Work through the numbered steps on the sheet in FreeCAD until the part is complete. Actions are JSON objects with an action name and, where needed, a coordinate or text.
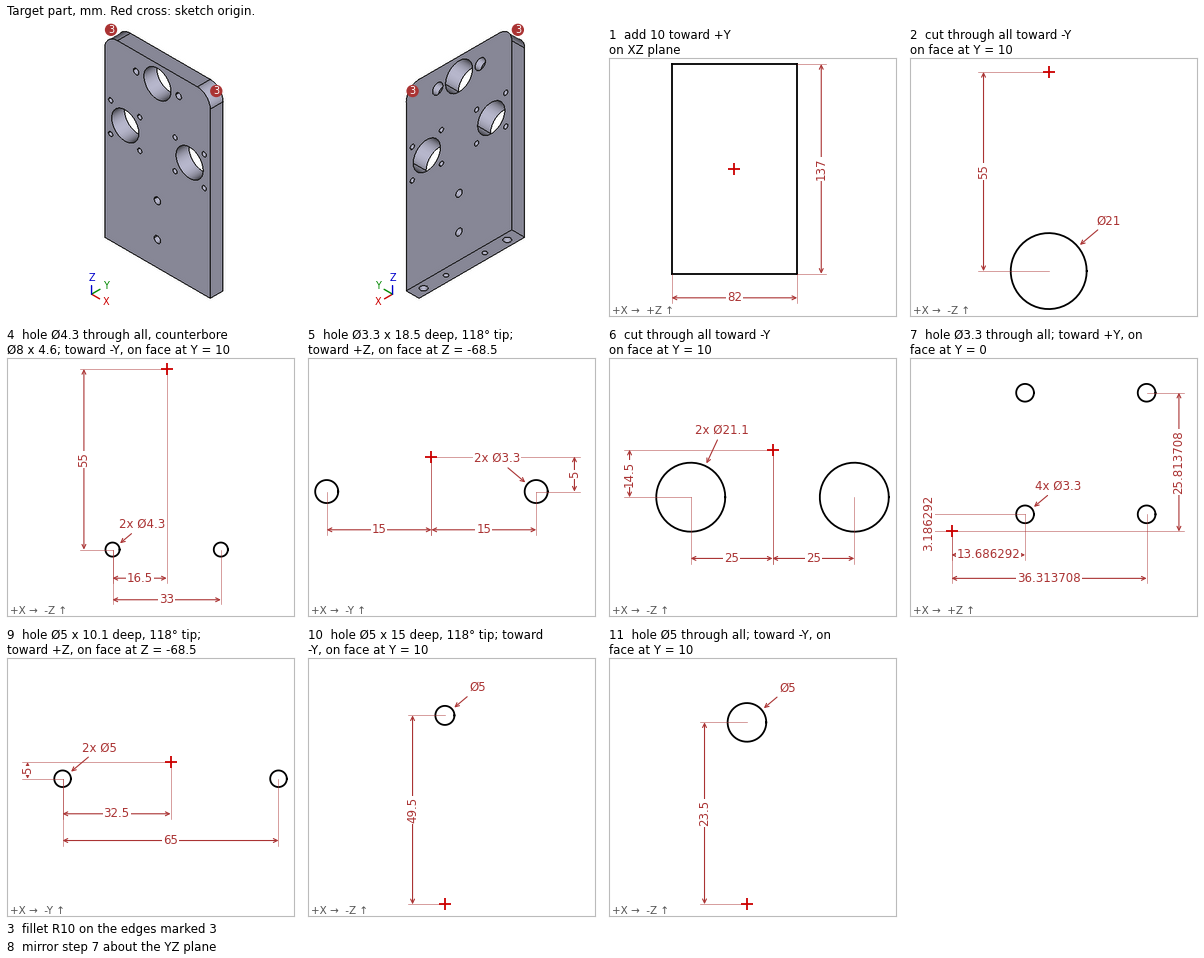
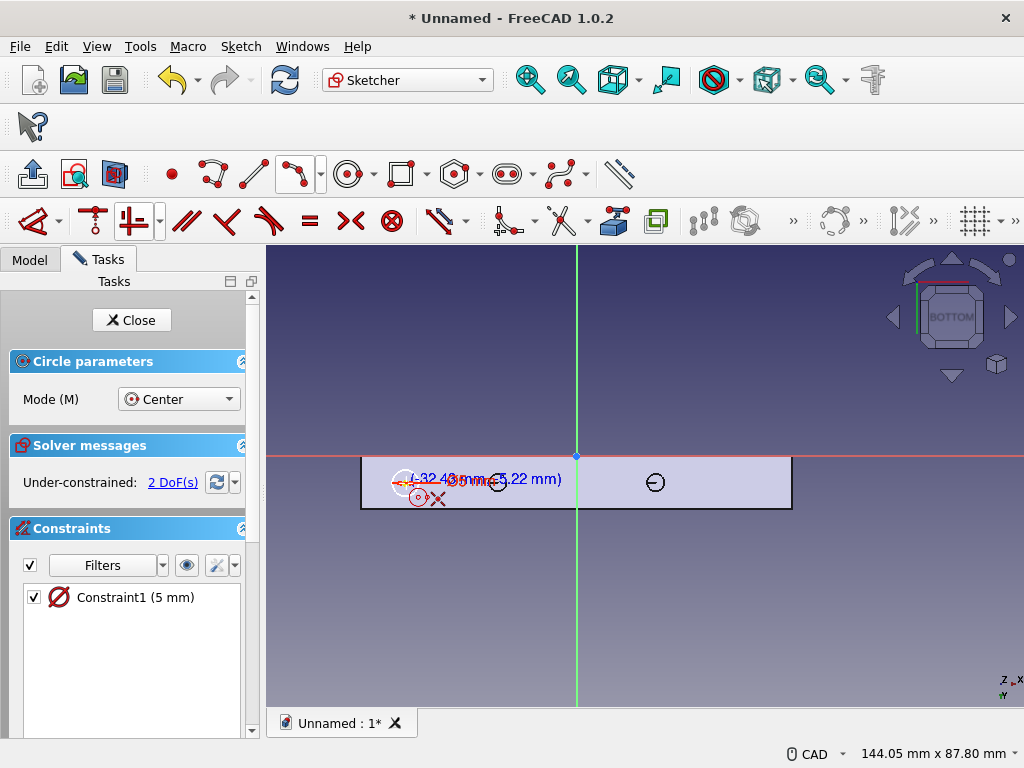
{"action": "scroll", "coordinate": [748, 483], "scroll_direction": "up", "scroll_amount": 3}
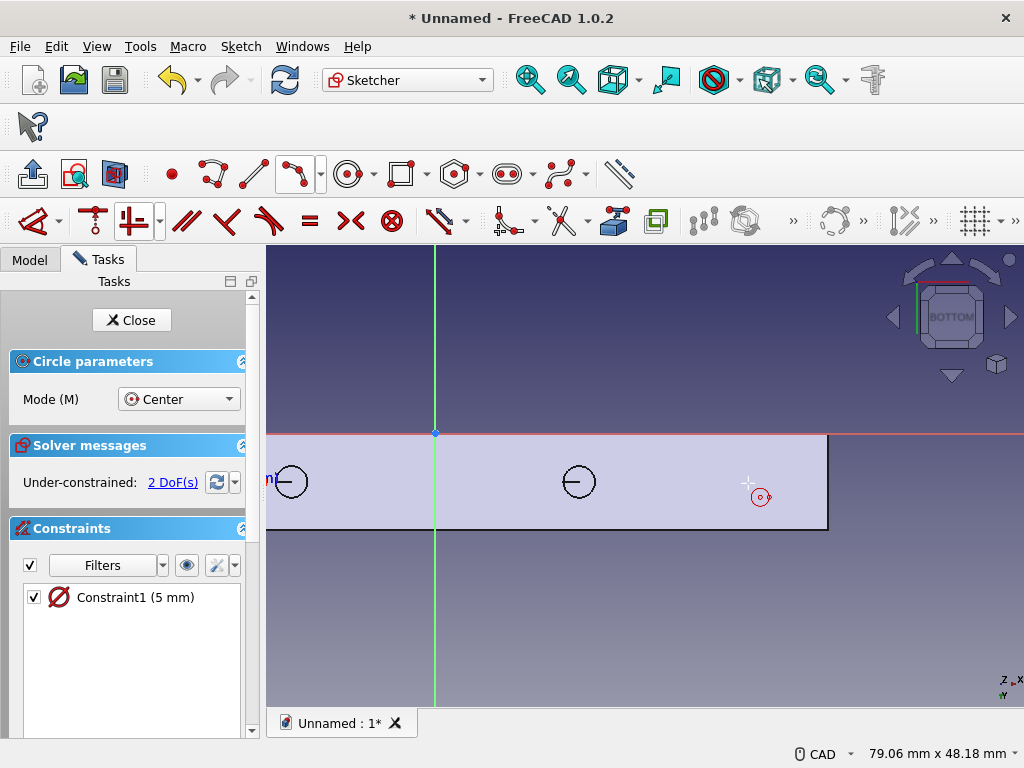
{"action": "left_click", "coordinate": [747, 482]}
{"action": "mouse_move", "coordinate": [764, 465]}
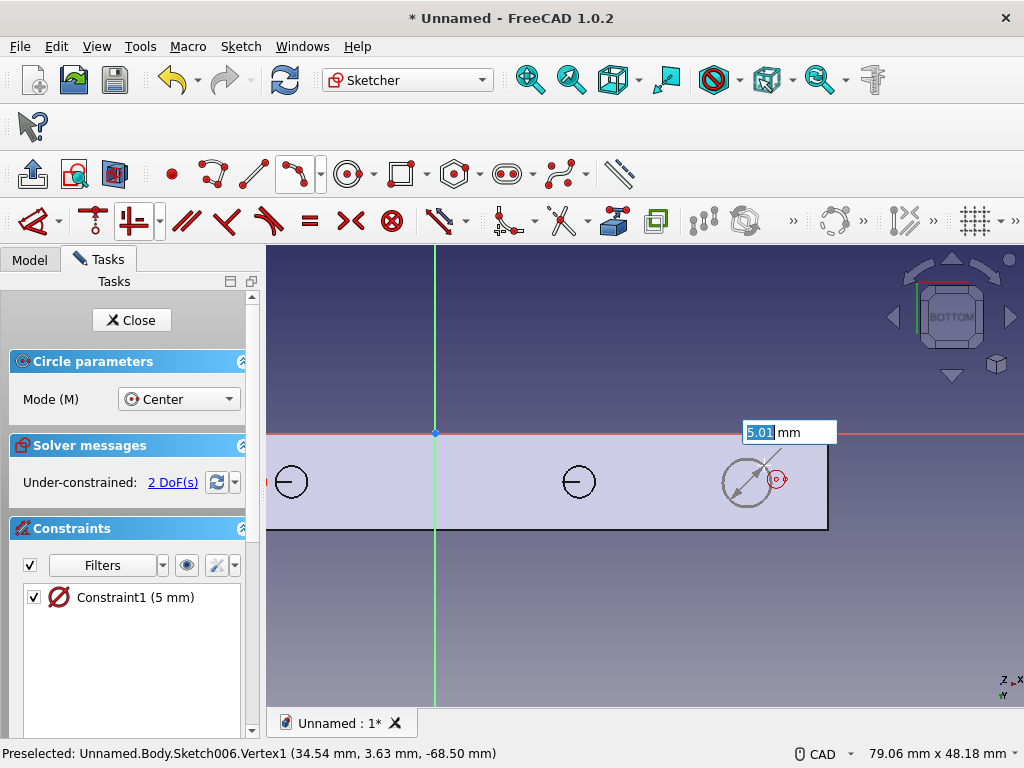
{"action": "type", "text": "5"}
{"action": "key", "text": "Return"}
{"action": "key", "text": "Escape"}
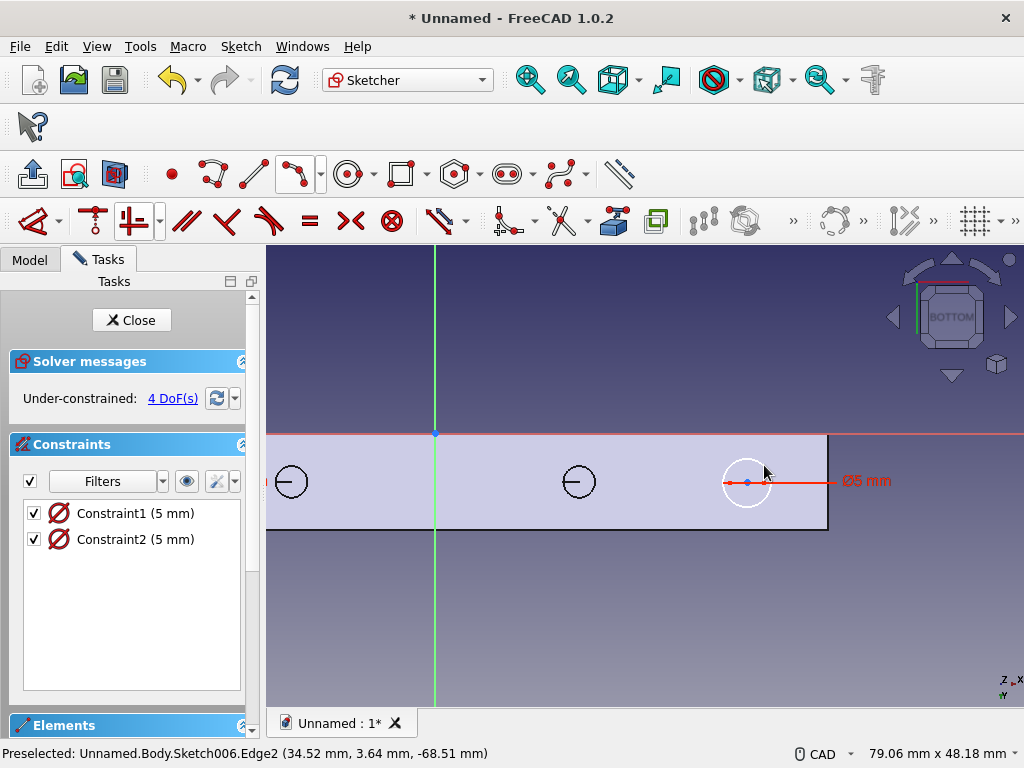
{"action": "scroll", "coordinate": [748, 483], "scroll_direction": "down", "scroll_amount": 3}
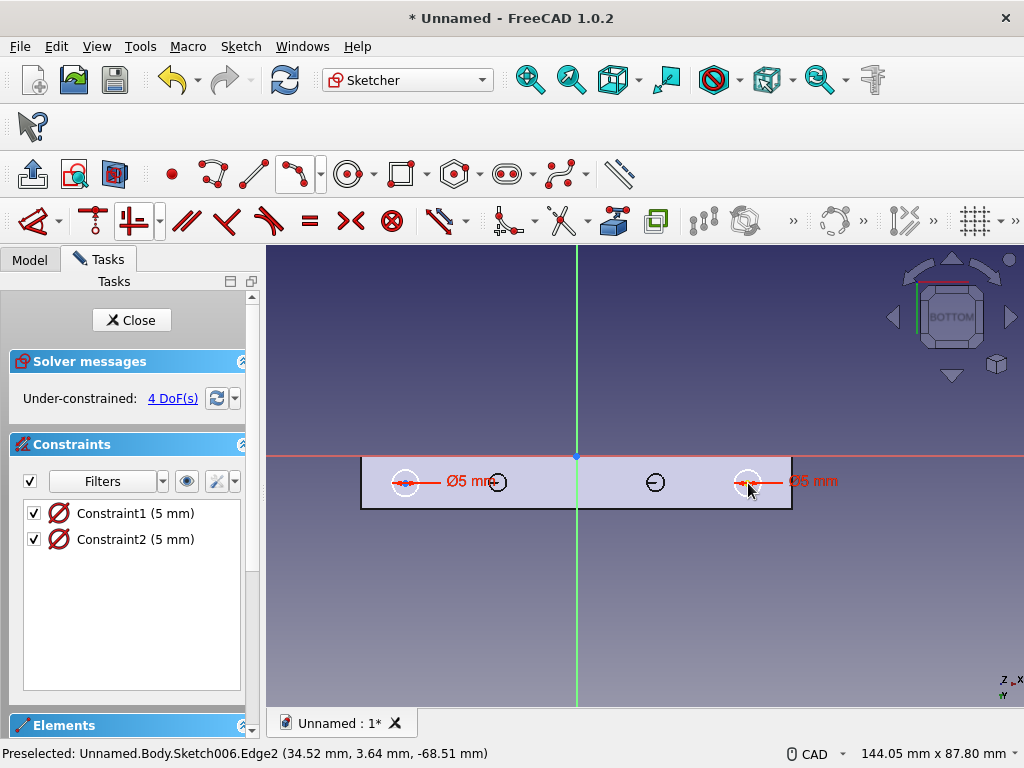
{"action": "left_click", "coordinate": [406, 483]}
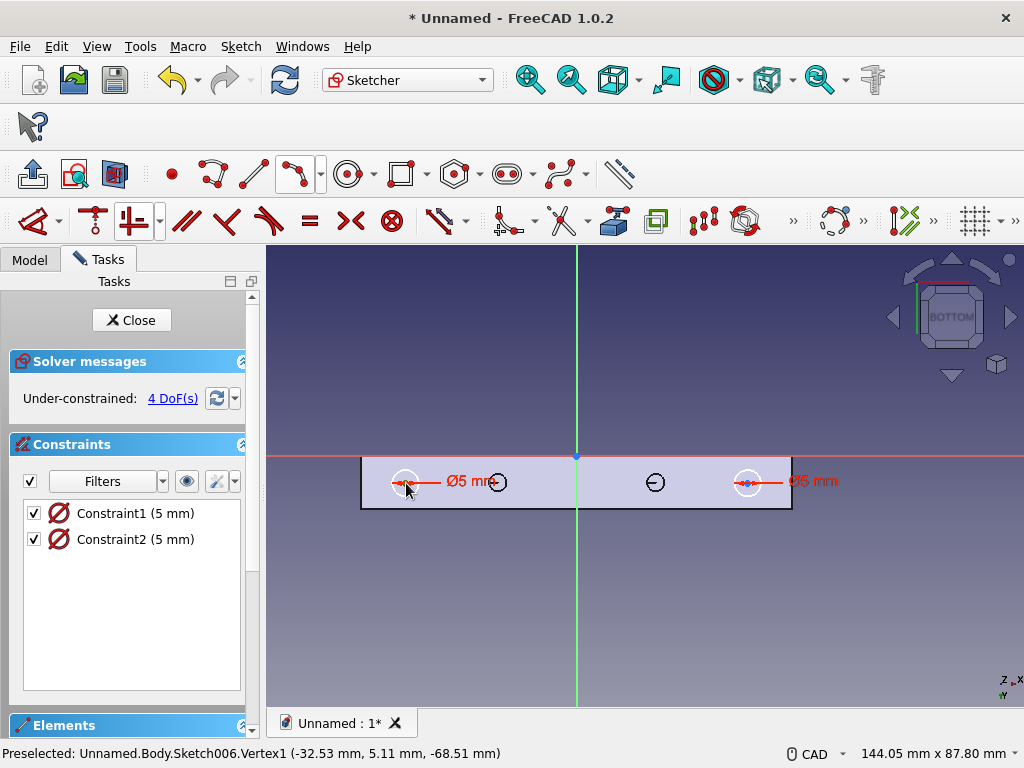
{"action": "left_click", "coordinate": [748, 483]}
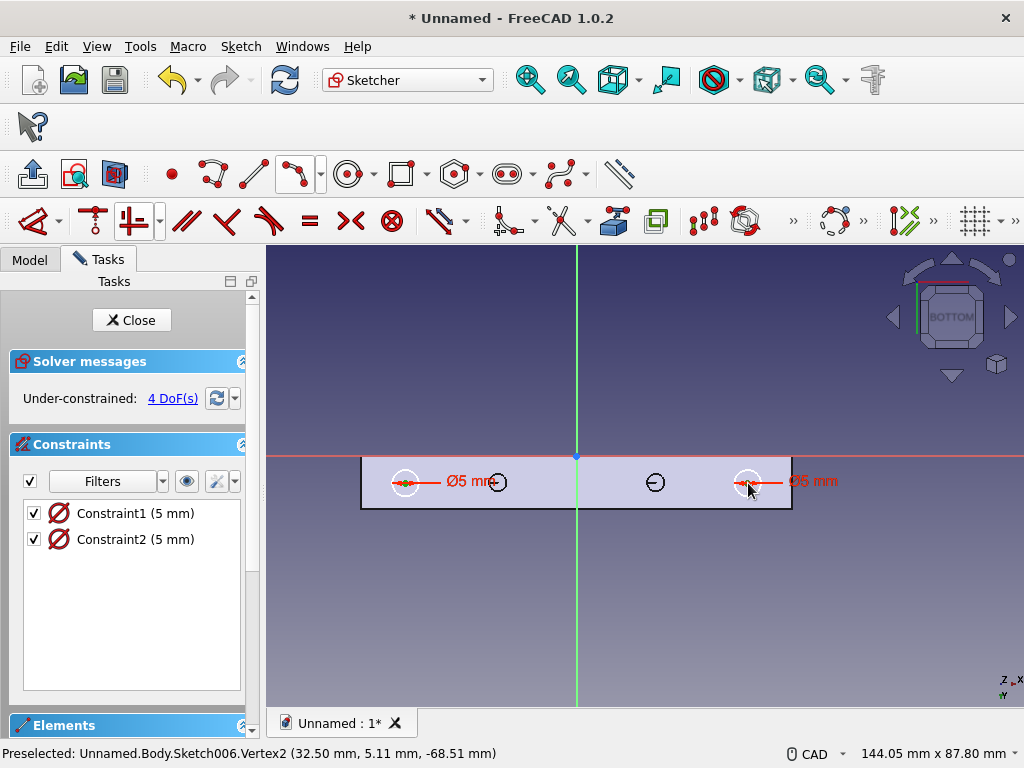
{"action": "key", "text": "h"}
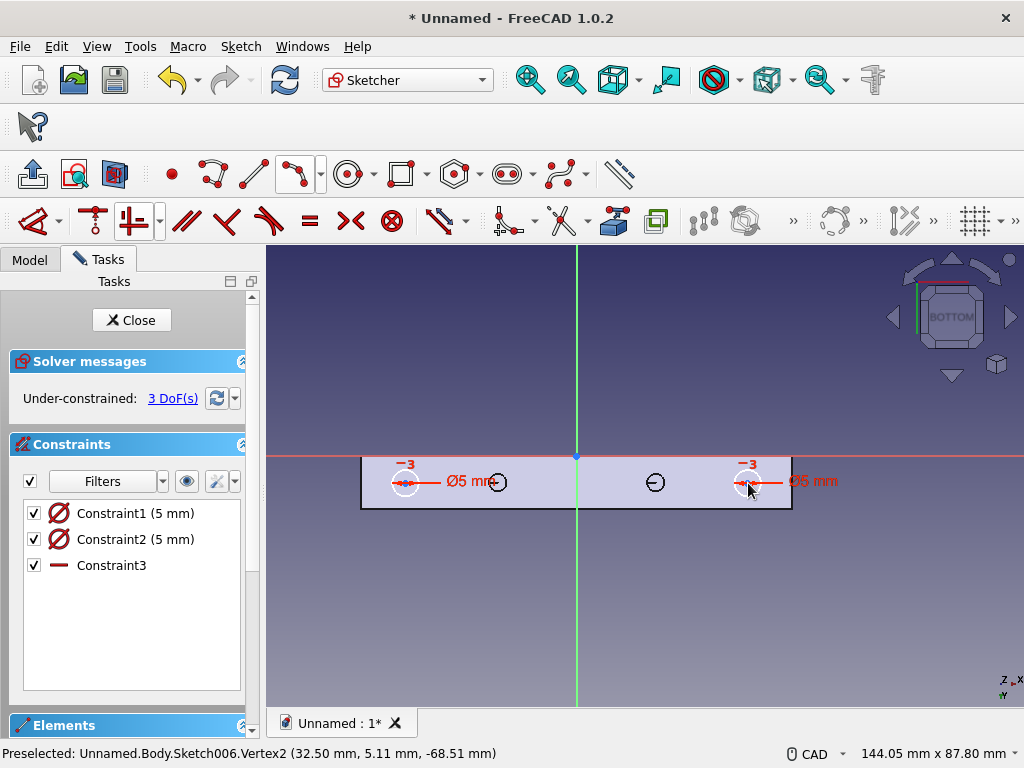
{"action": "left_click", "coordinate": [32, 222]}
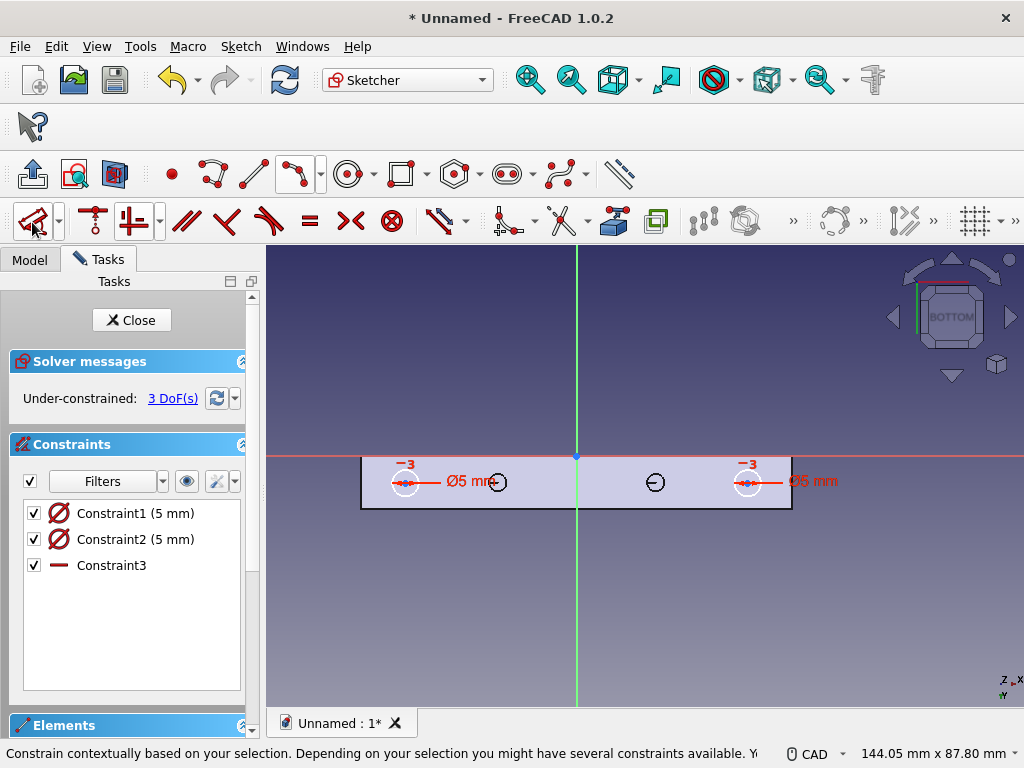
{"action": "scroll", "coordinate": [406, 483], "scroll_direction": "up", "scroll_amount": 3}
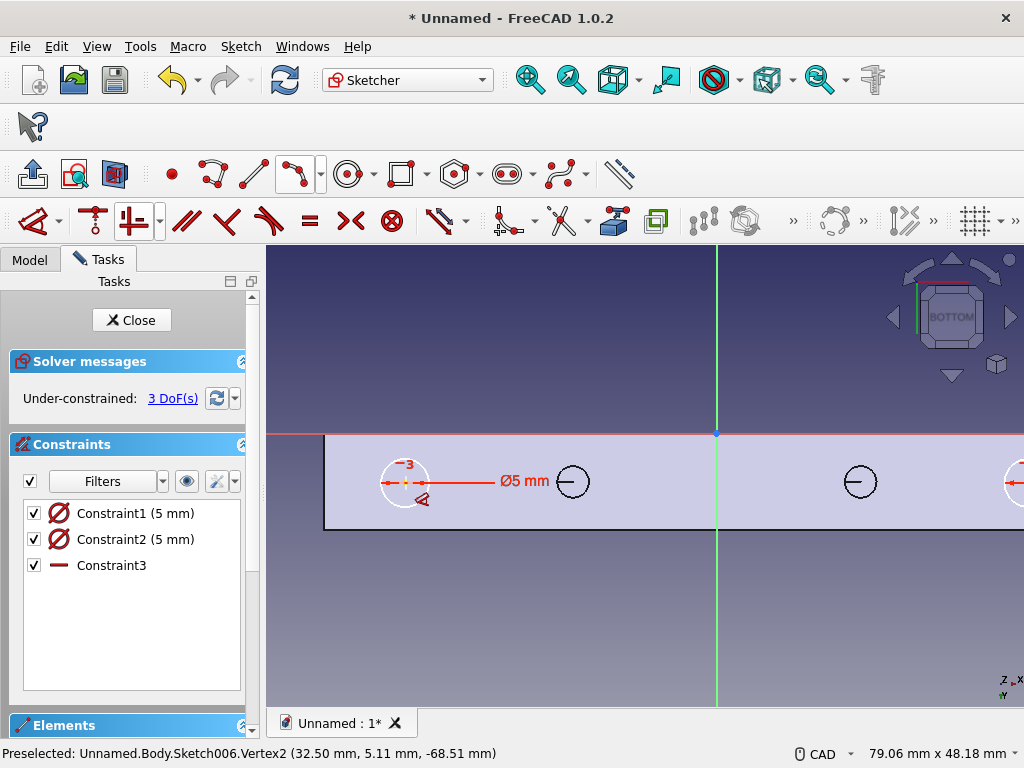
{"action": "left_click", "coordinate": [405, 483]}
{"action": "left_click", "coordinate": [371, 458]}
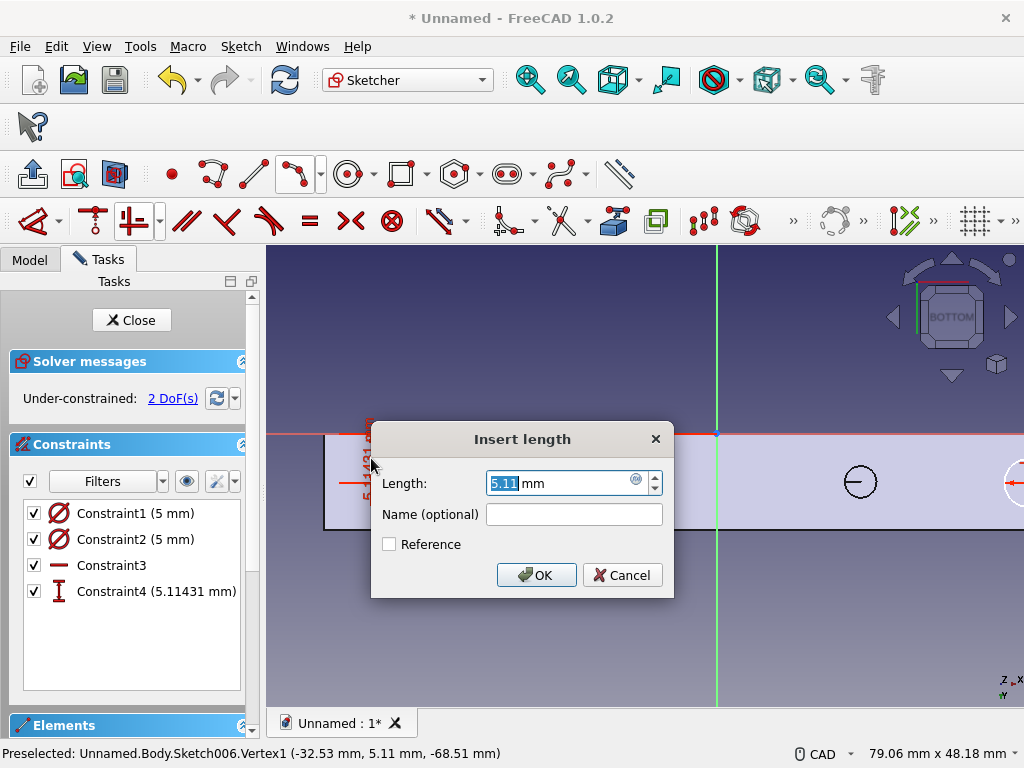
{"action": "type", "text": "5"}
{"action": "key", "text": "Return"}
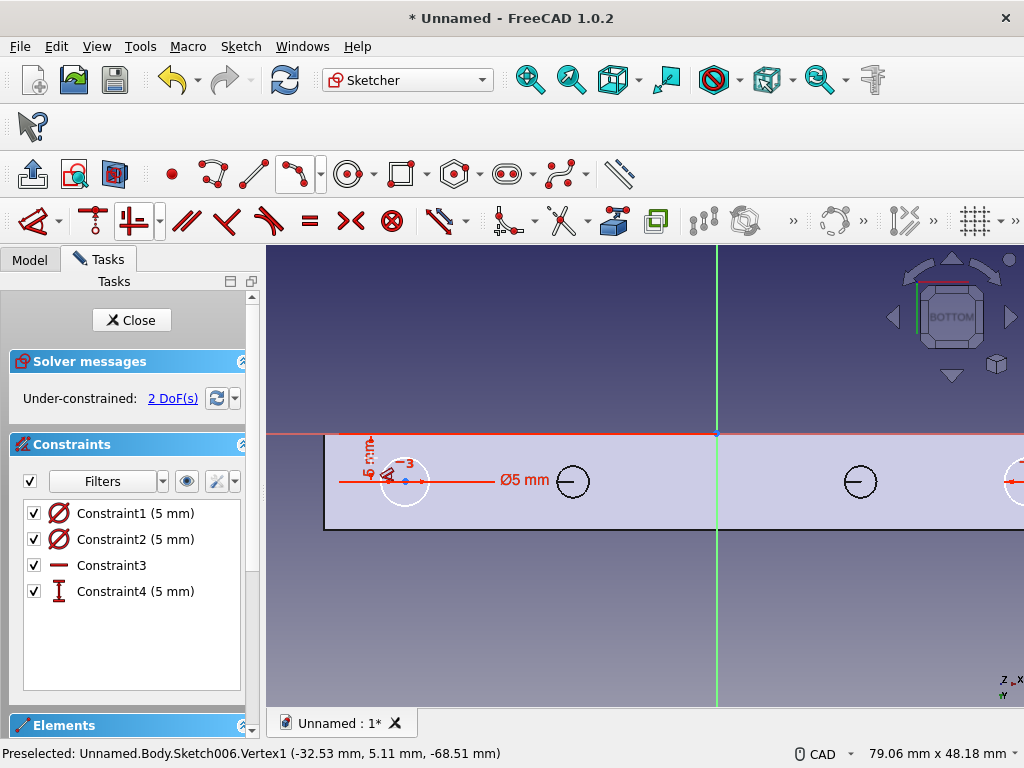
{"action": "left_click", "coordinate": [405, 482]}